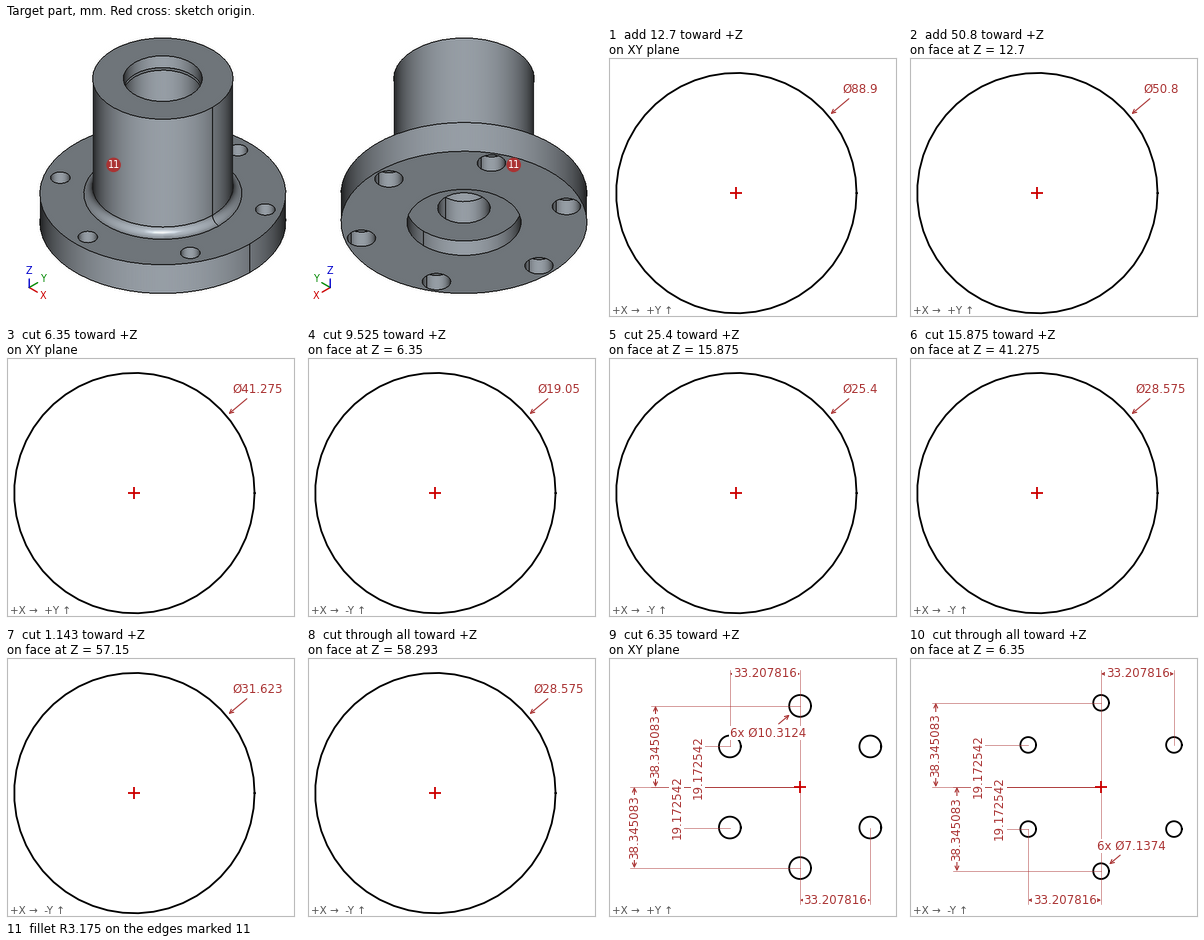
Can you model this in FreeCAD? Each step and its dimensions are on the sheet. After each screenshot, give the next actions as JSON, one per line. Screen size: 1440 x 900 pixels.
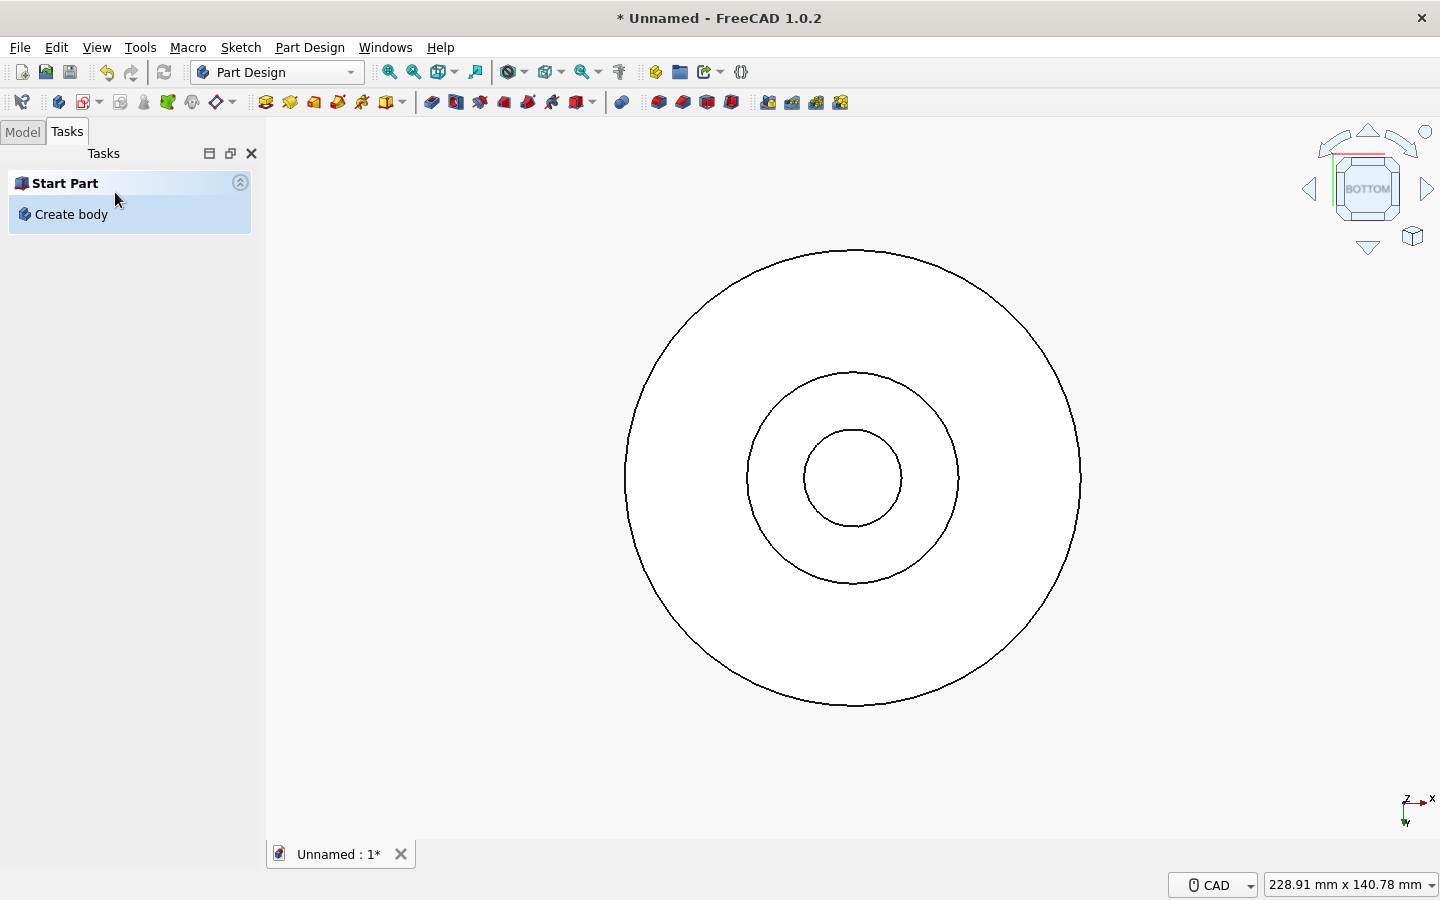
{"action": "left_click", "coordinate": [853, 477]}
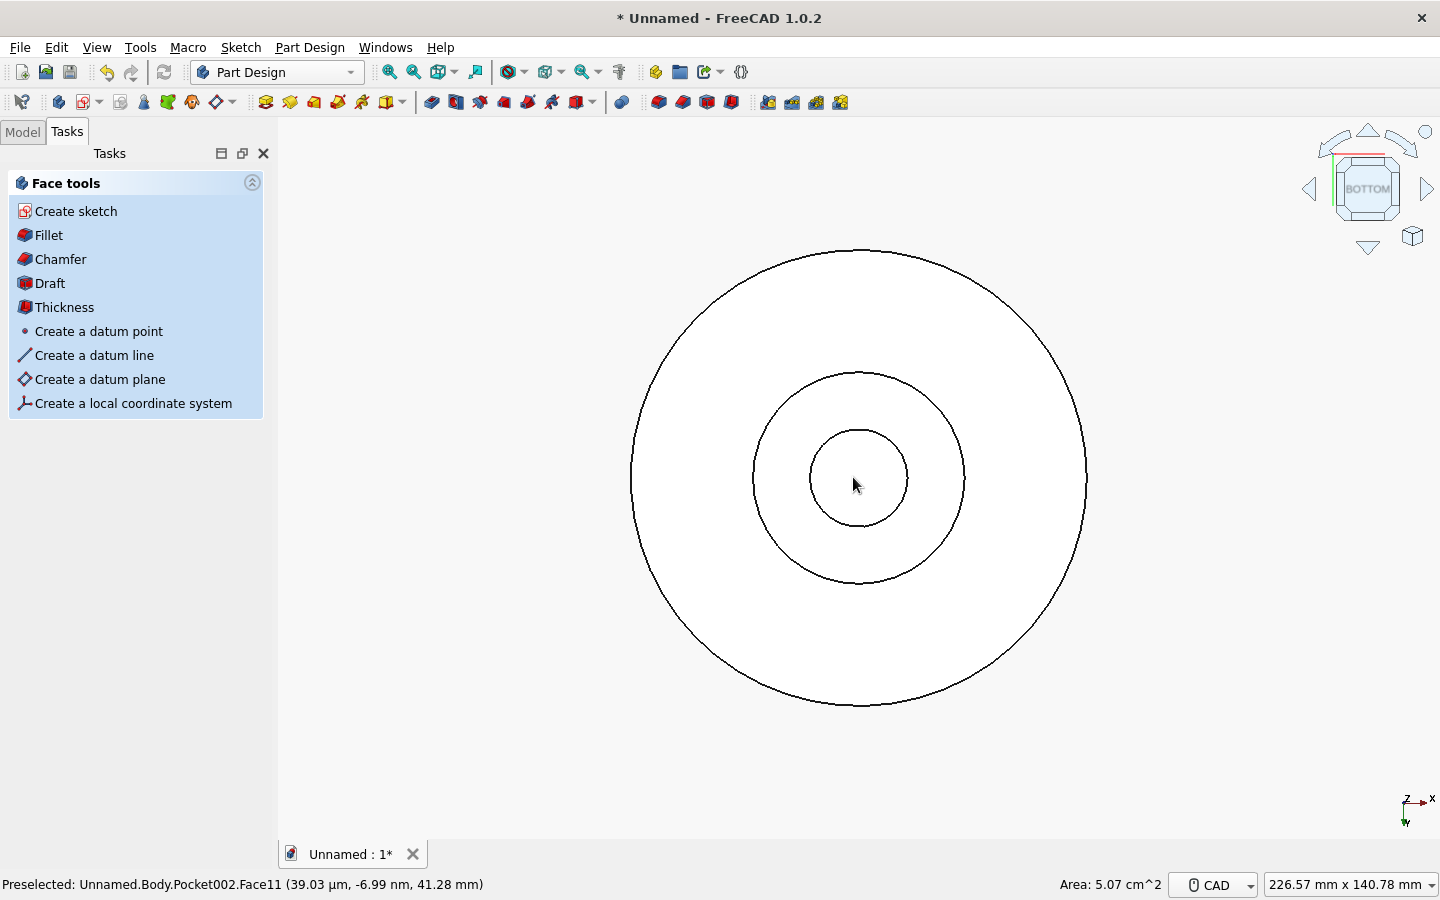
{"action": "left_click", "coordinate": [84, 102]}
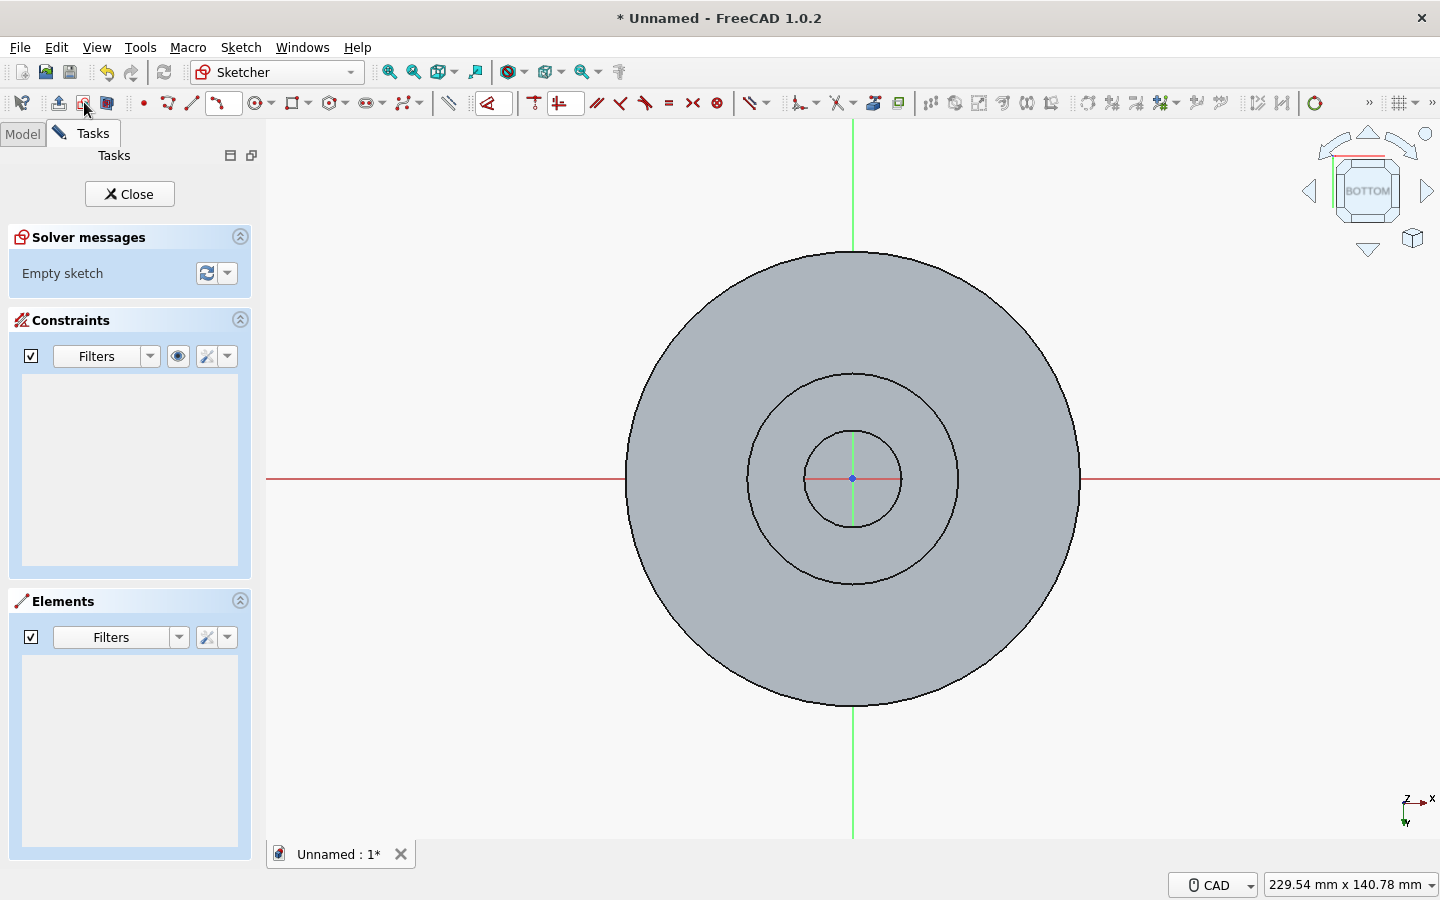
{"action": "key", "text": "q s"}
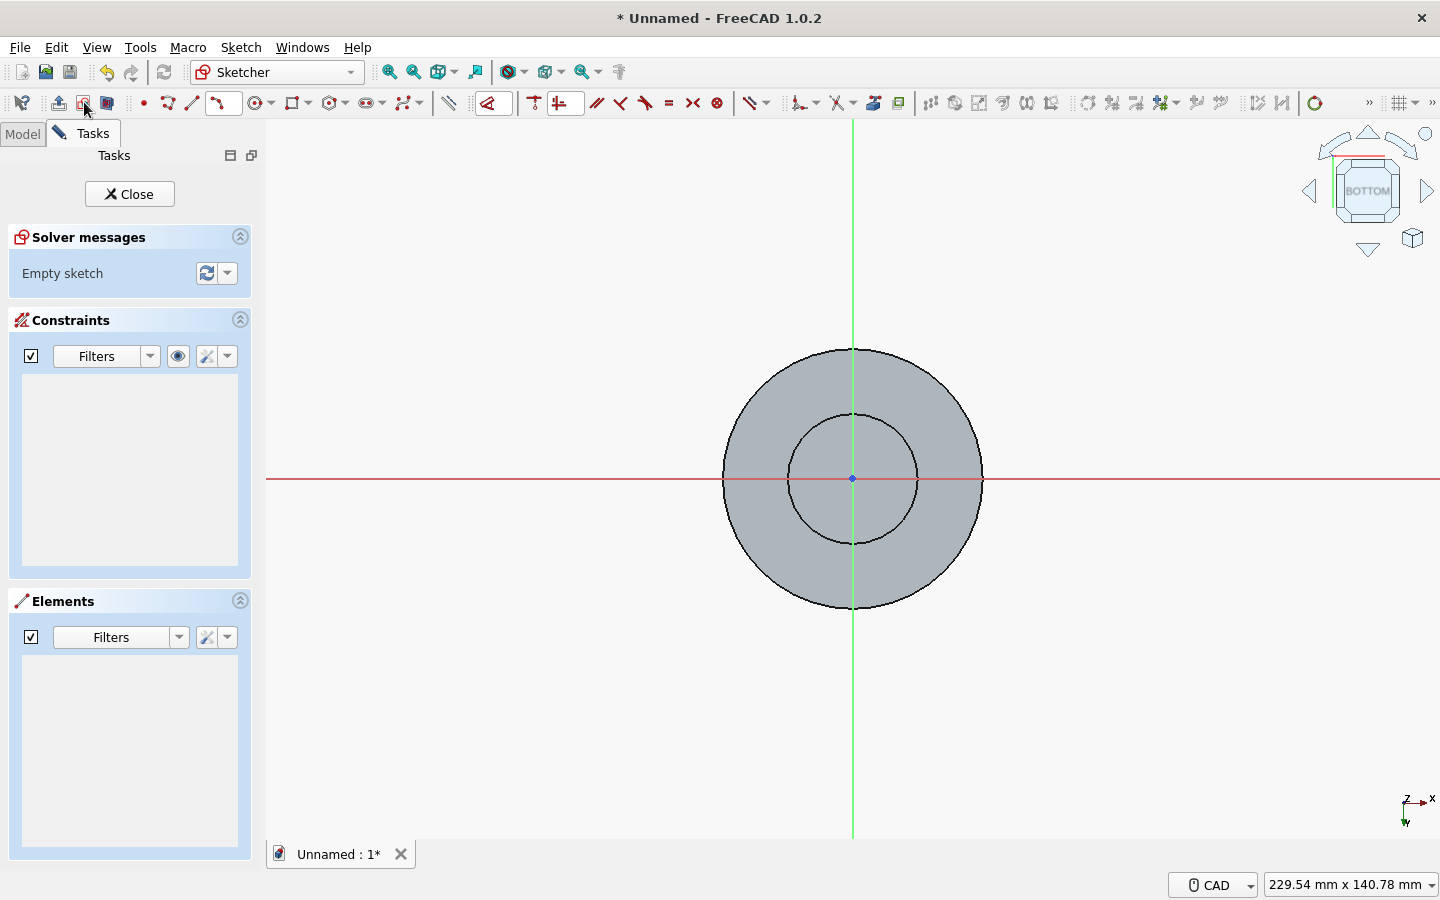
{"action": "scroll", "coordinate": [882, 479], "scroll_direction": "up", "scroll_amount": 6}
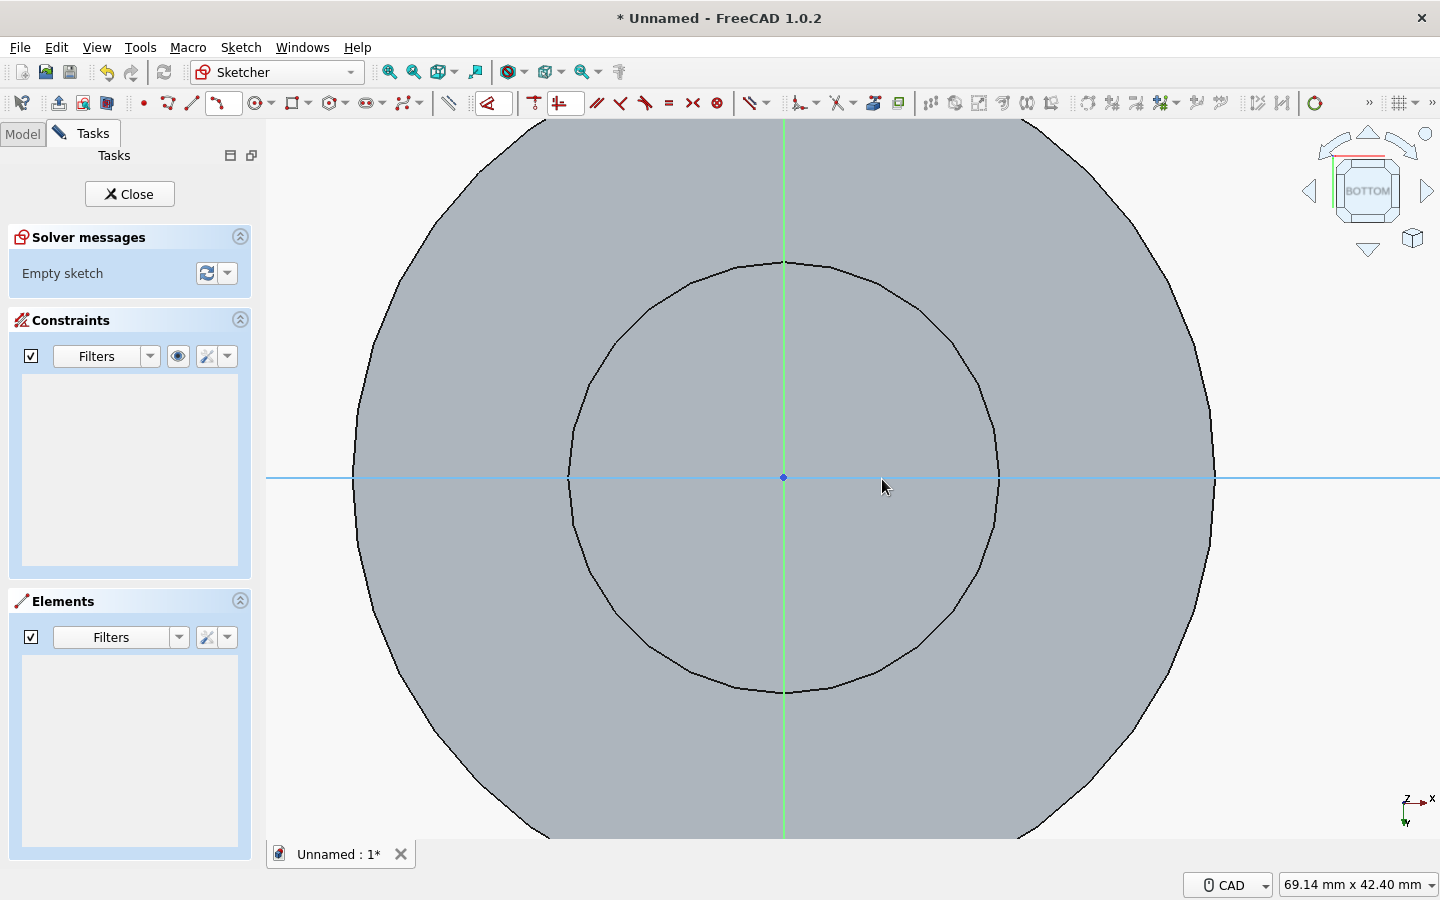
{"action": "key", "text": "g c"}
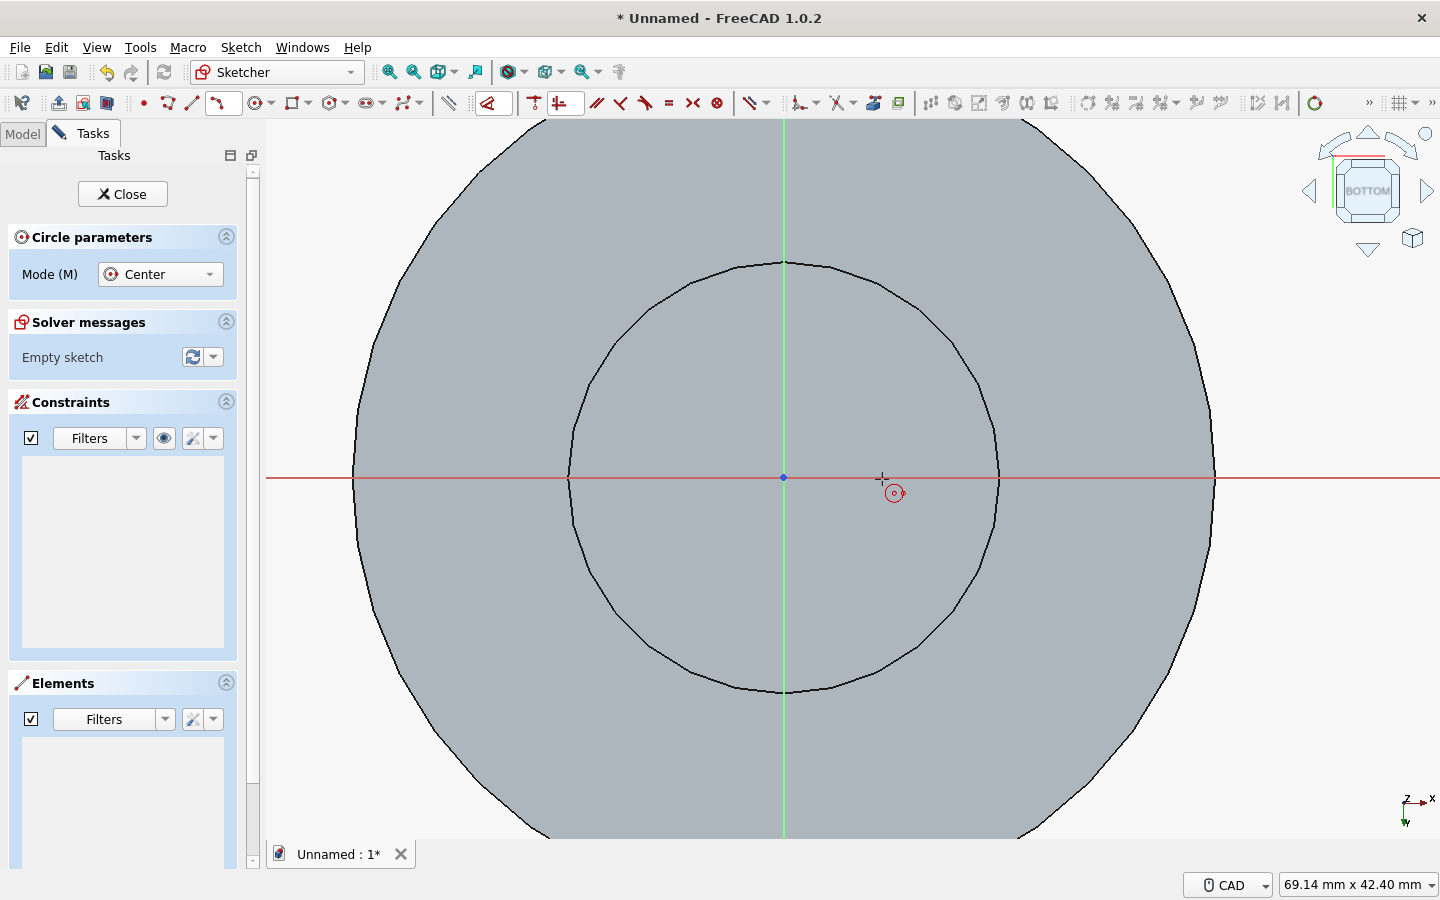
{"action": "left_click", "coordinate": [784, 478]}
{"action": "mouse_move", "coordinate": [955, 306]}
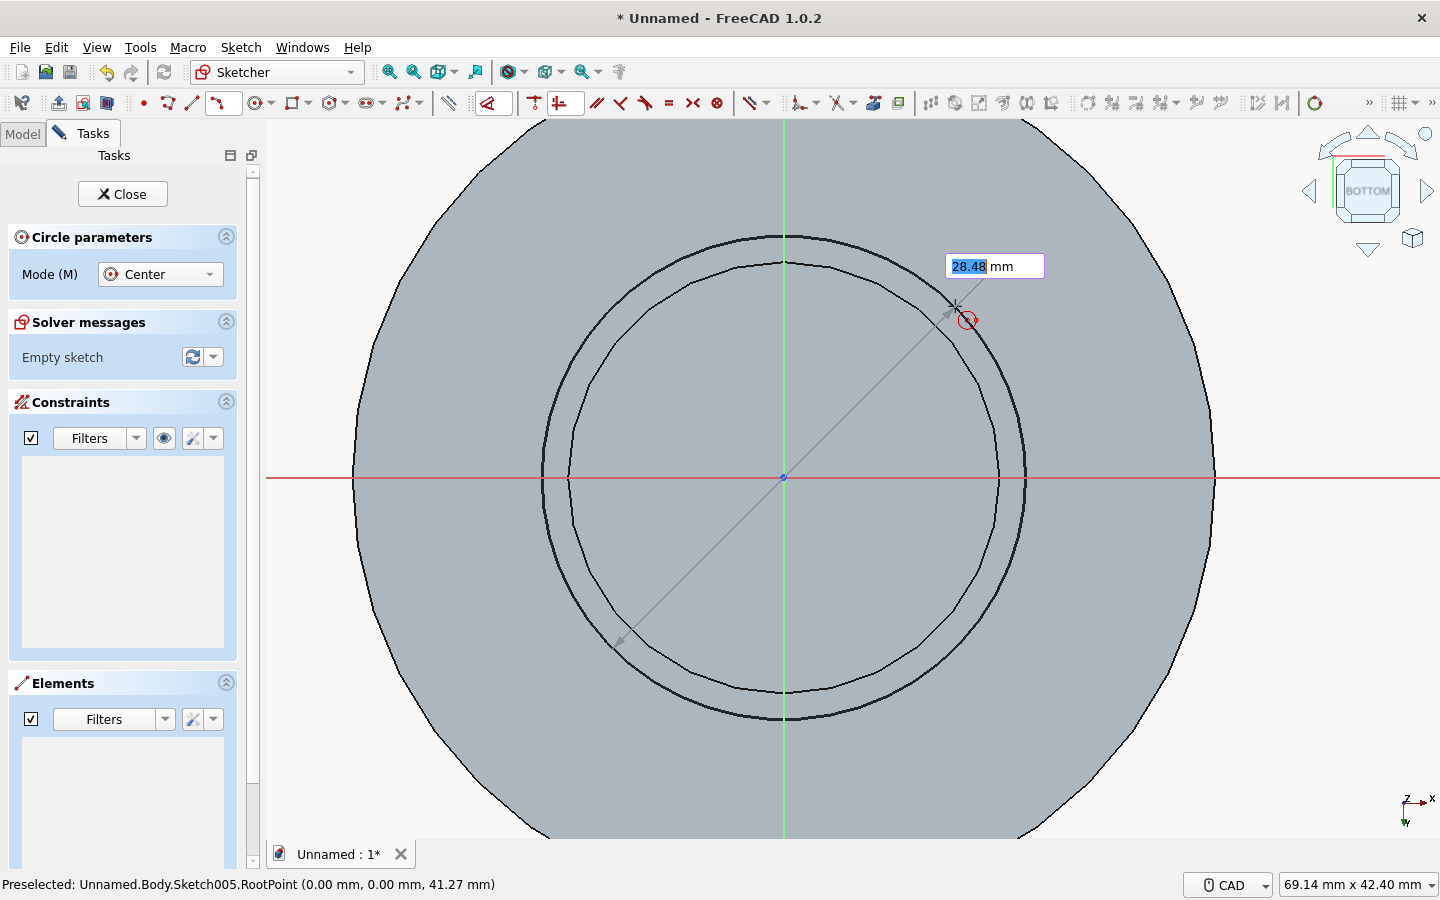
{"action": "type", "text": "28.575"}
{"action": "key", "text": "Return"}
{"action": "key", "text": "Escape"}